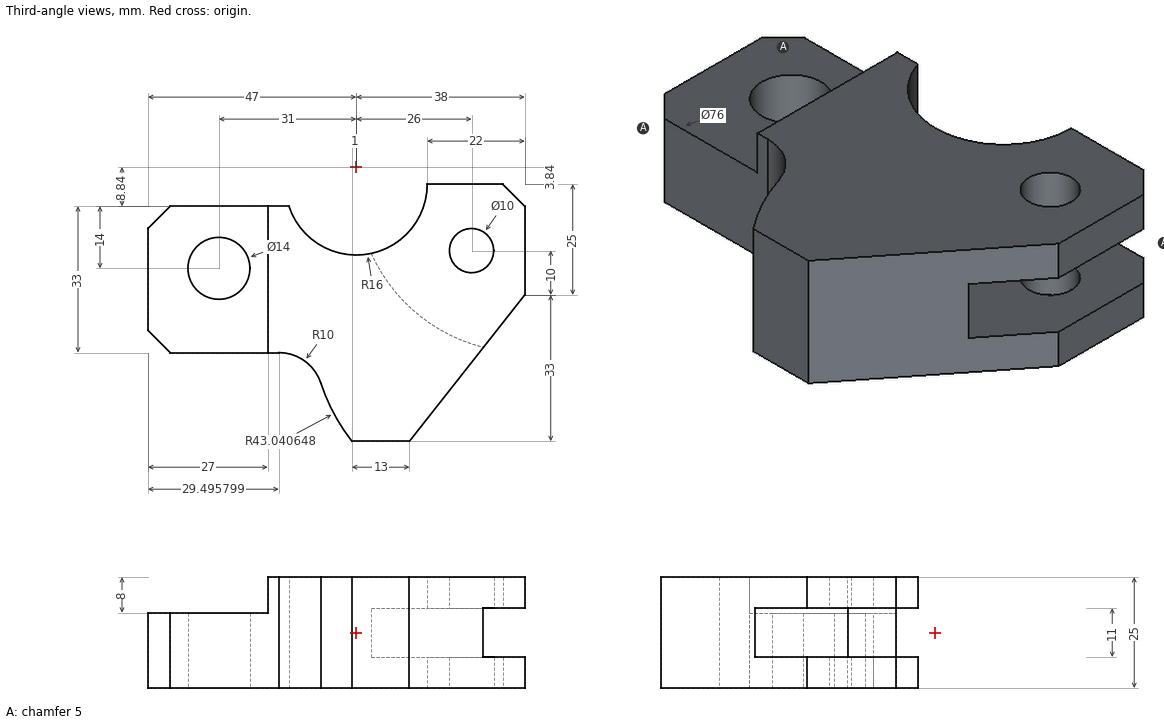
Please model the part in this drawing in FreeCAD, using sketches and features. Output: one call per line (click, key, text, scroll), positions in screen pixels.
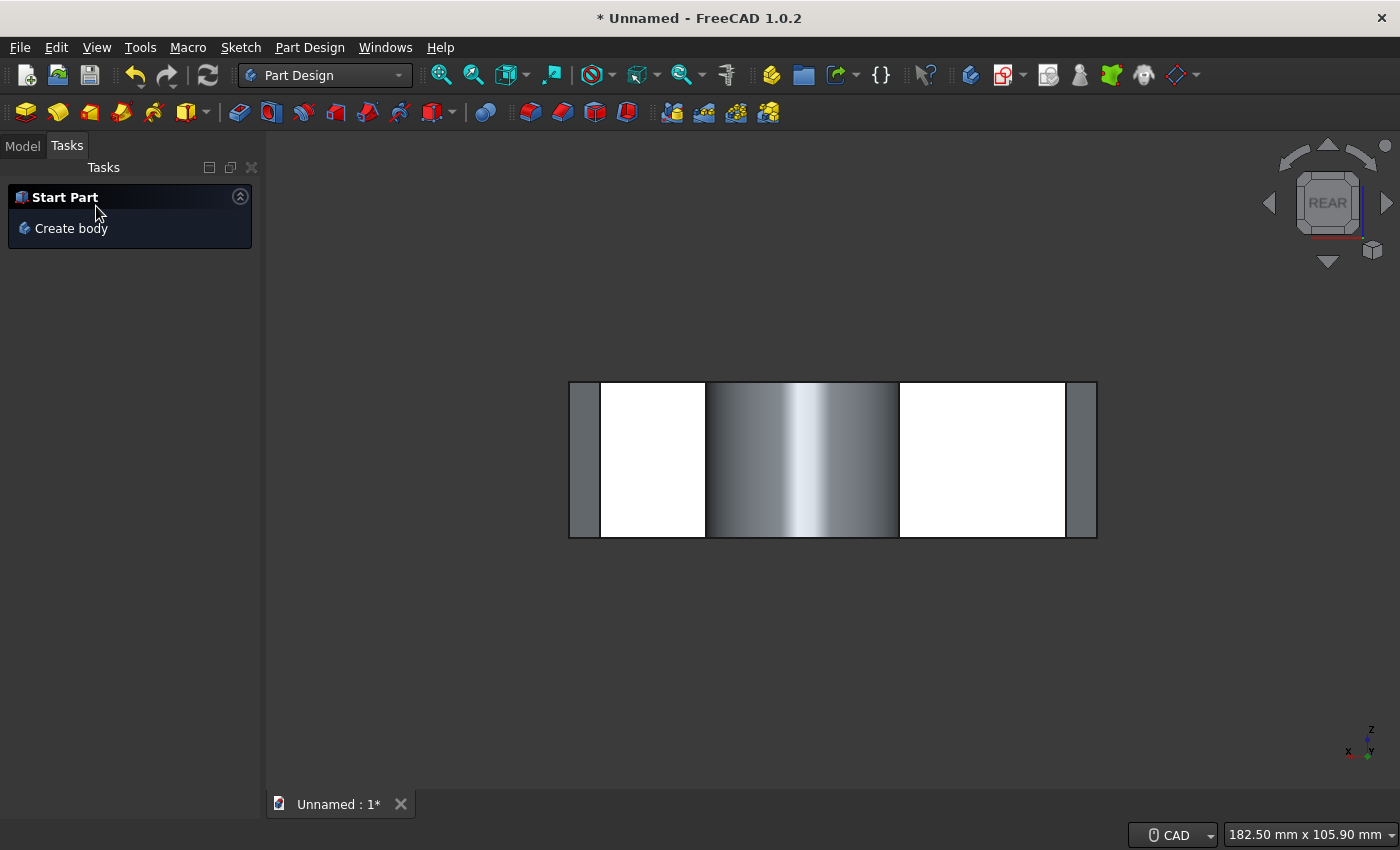
key(0)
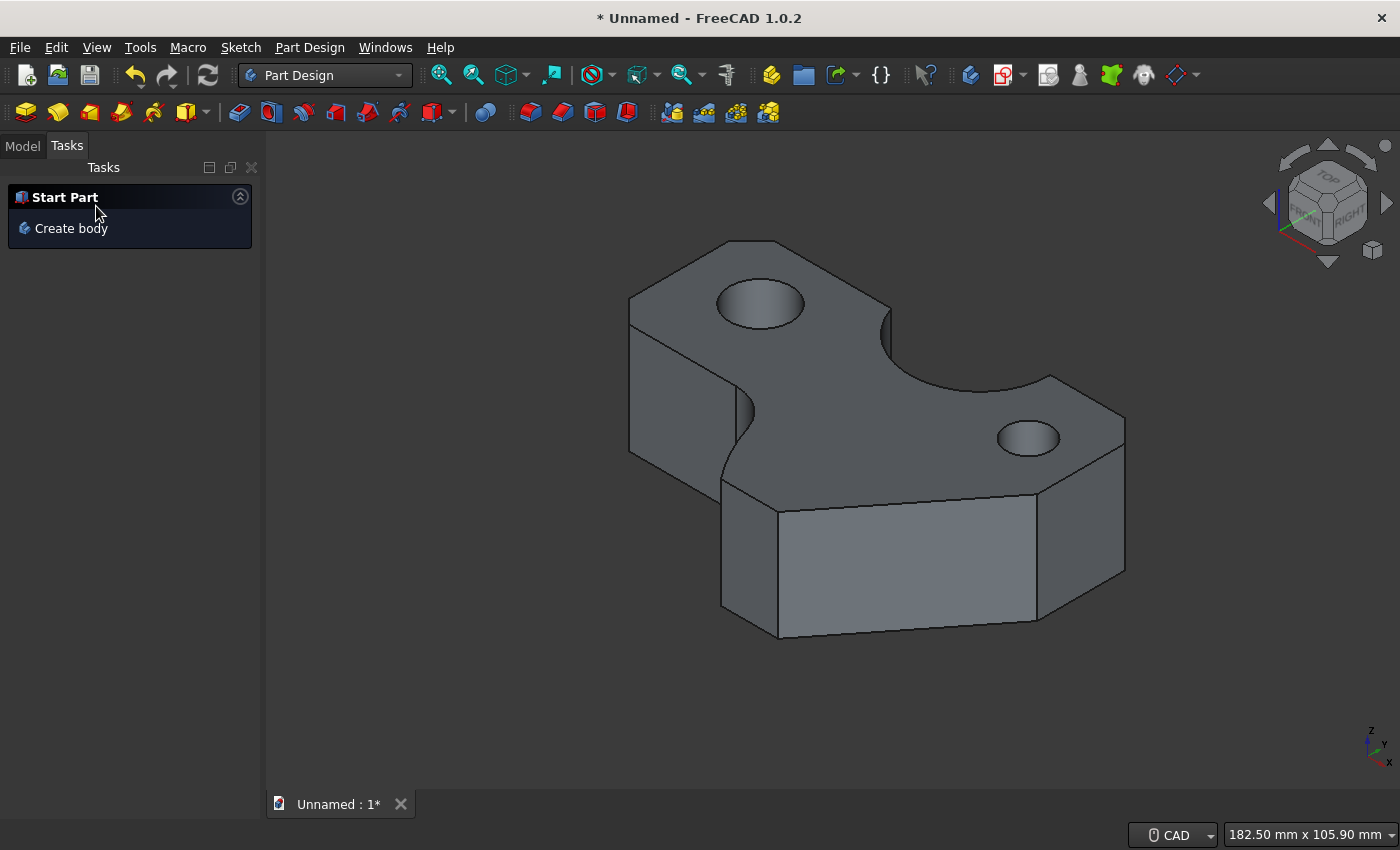
click(850, 447)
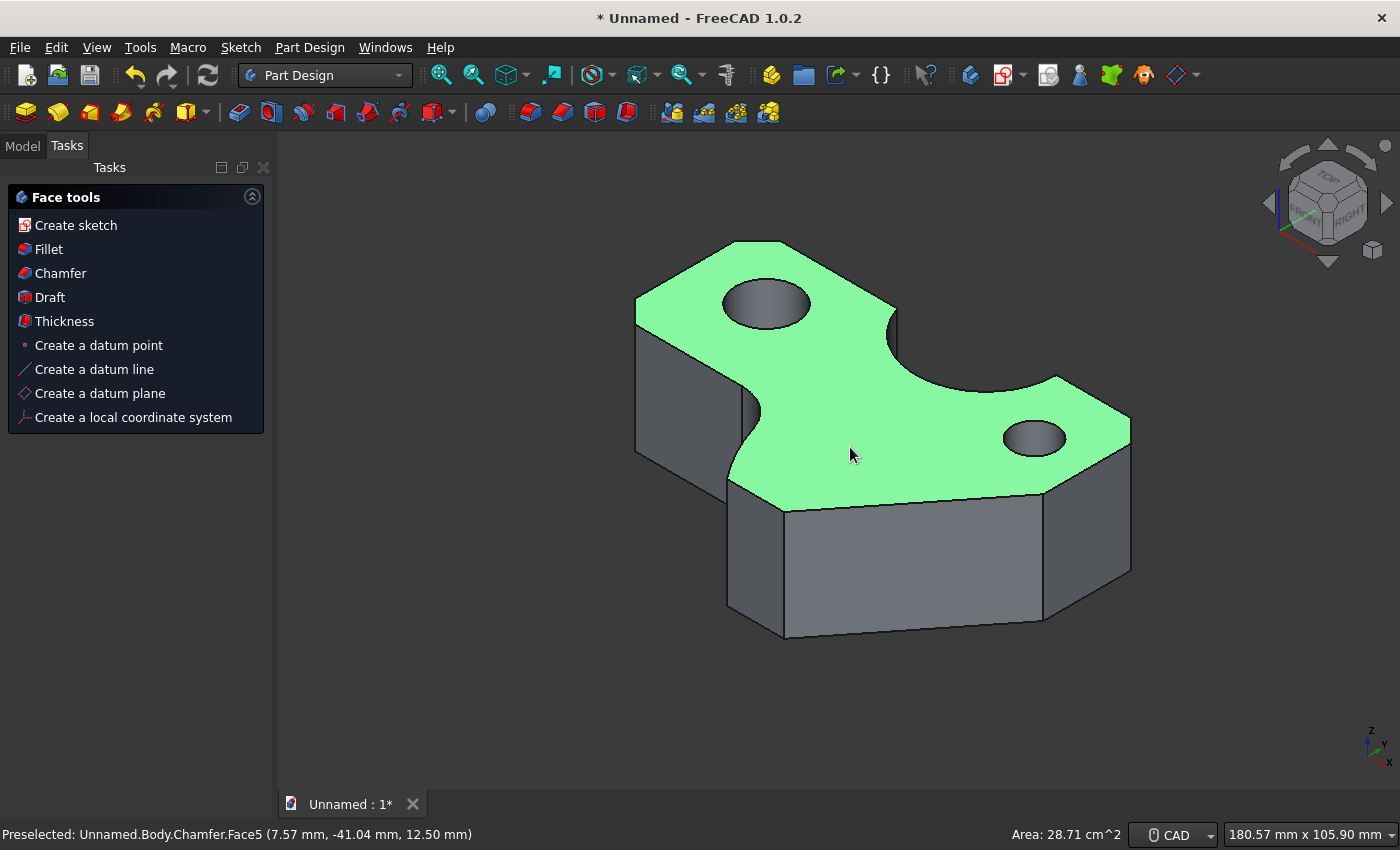
click(1004, 76)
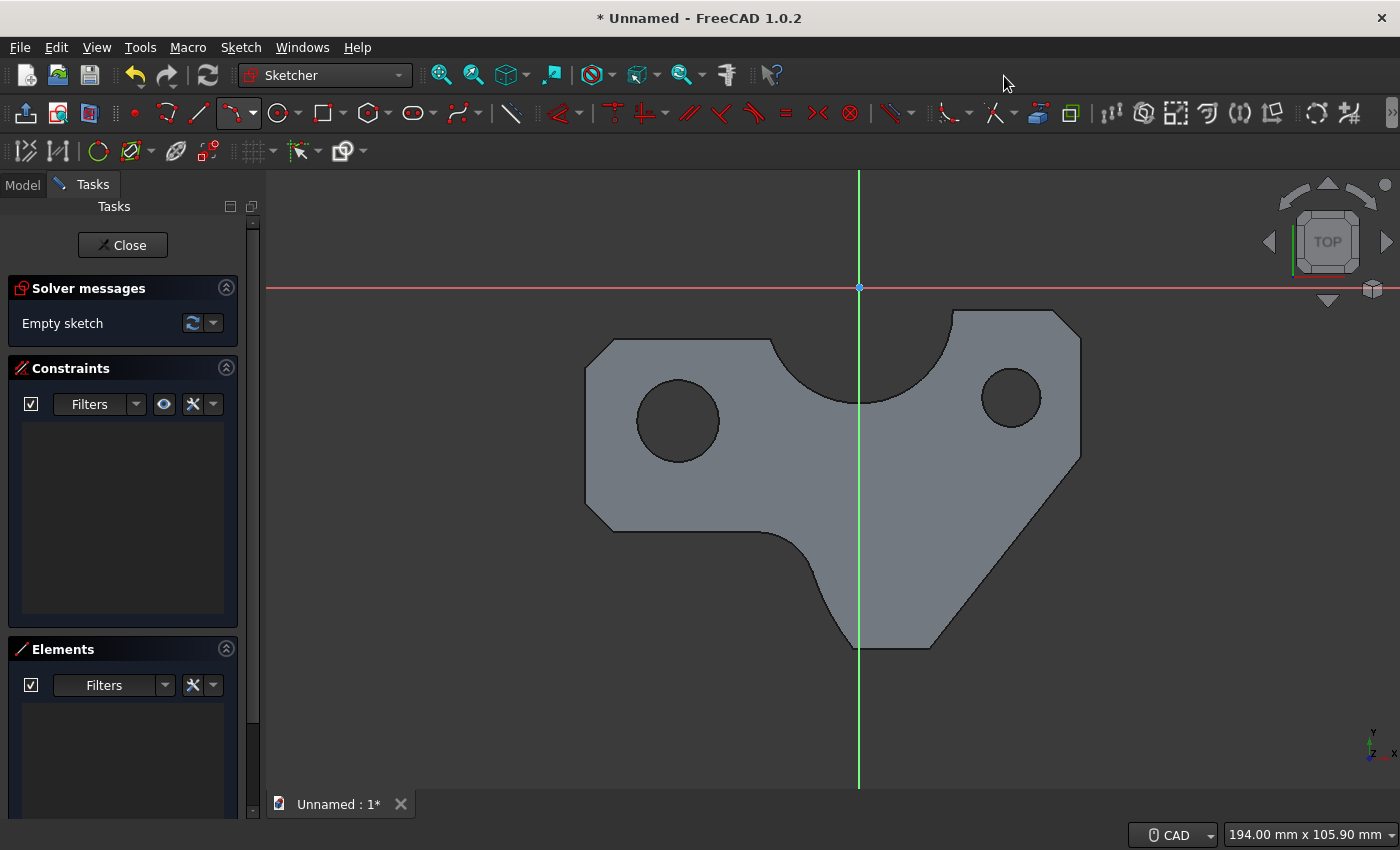
scroll(635, 268, up, 2)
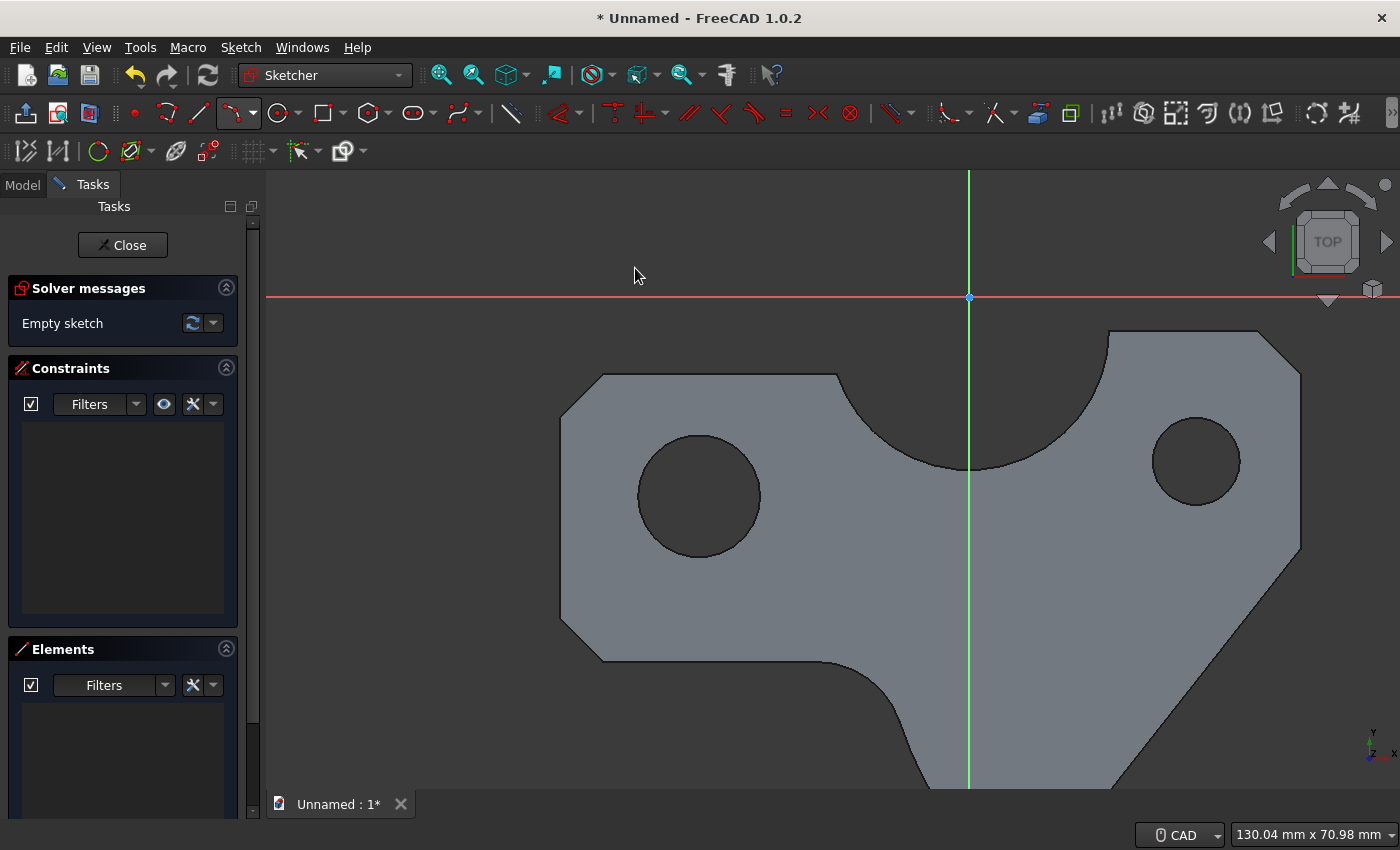
key(g)
key(r)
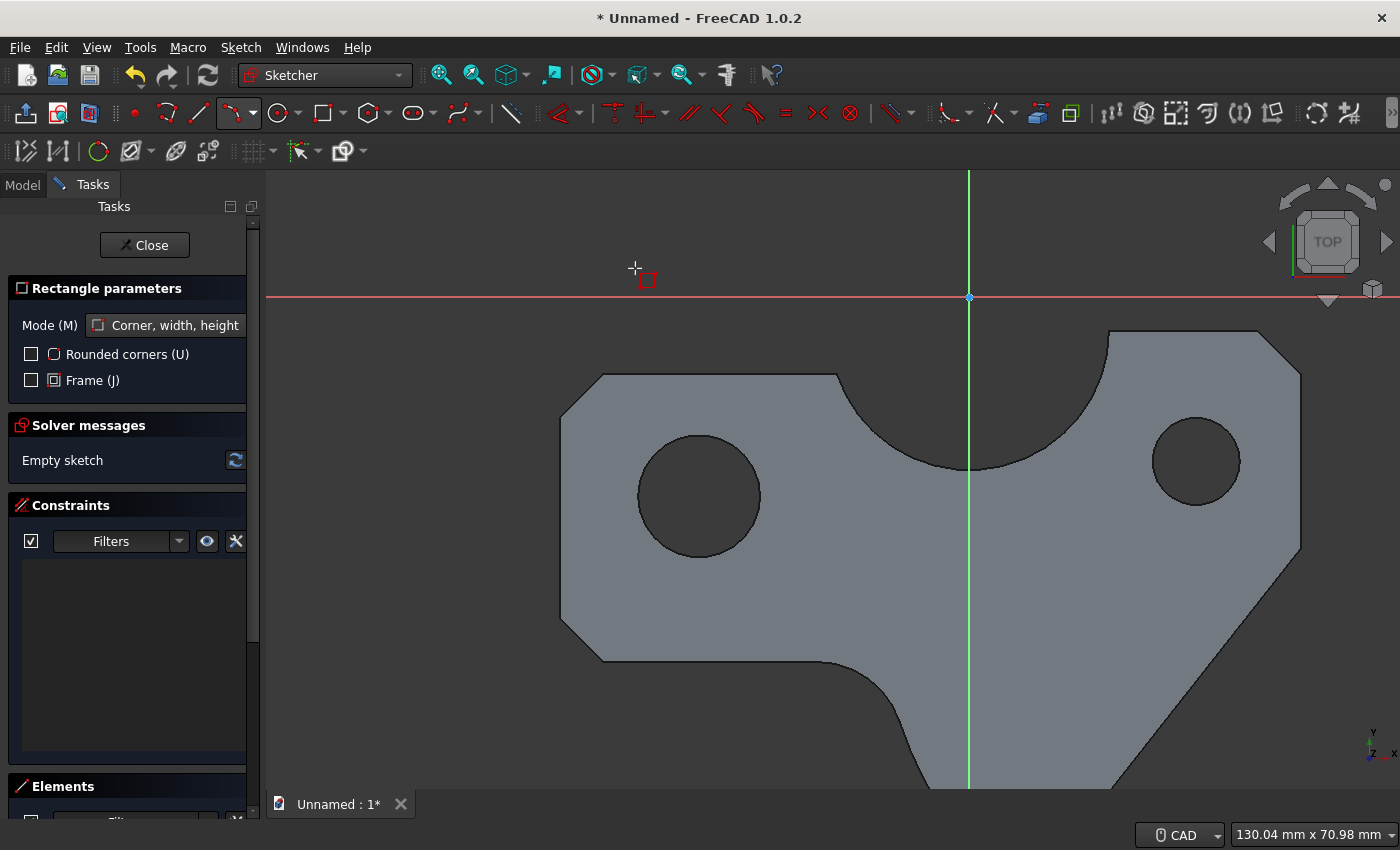
click(560, 374)
move(795, 662)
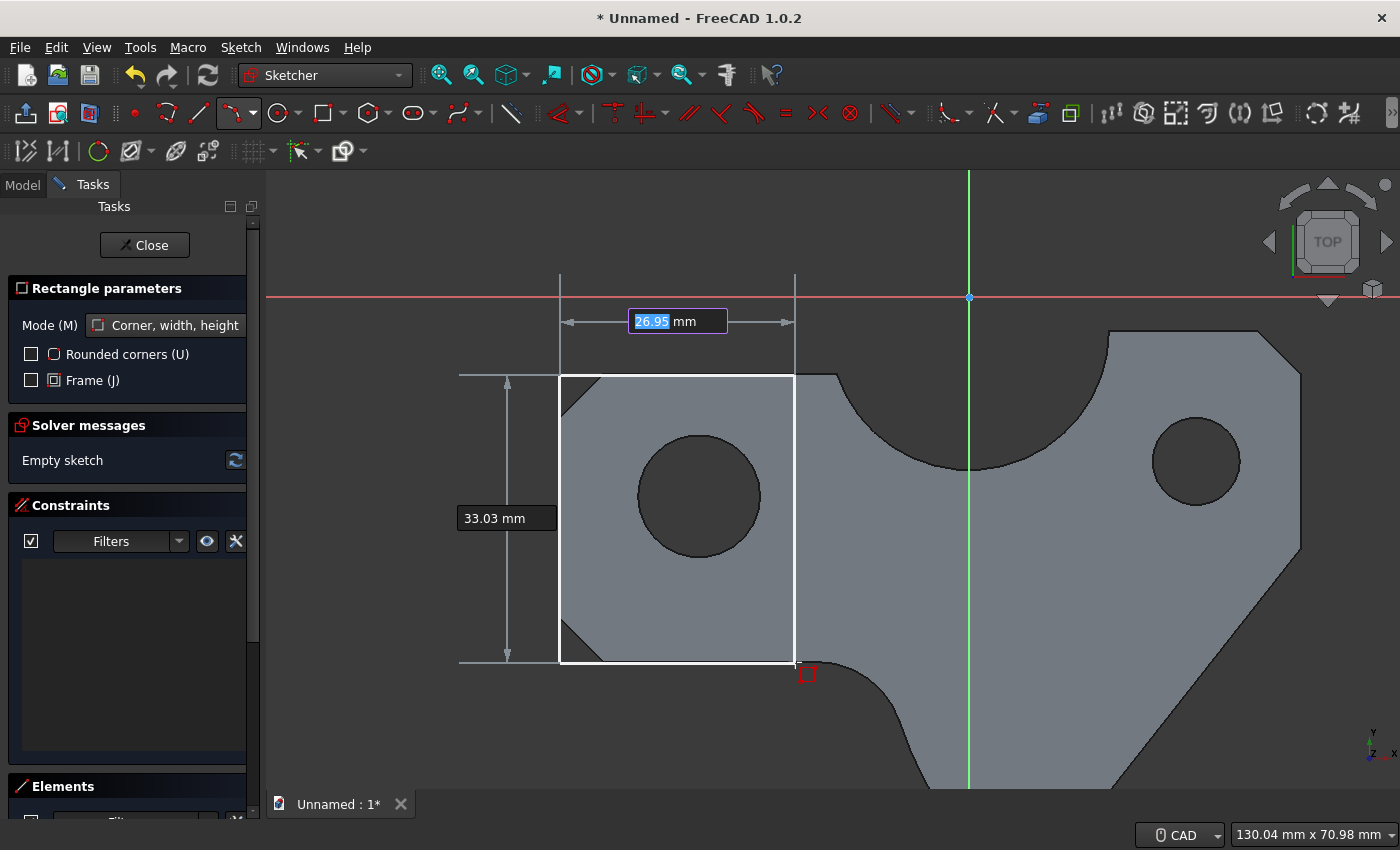
text(27)
key(Tab)
text(33)
key(Return)
key(Escape)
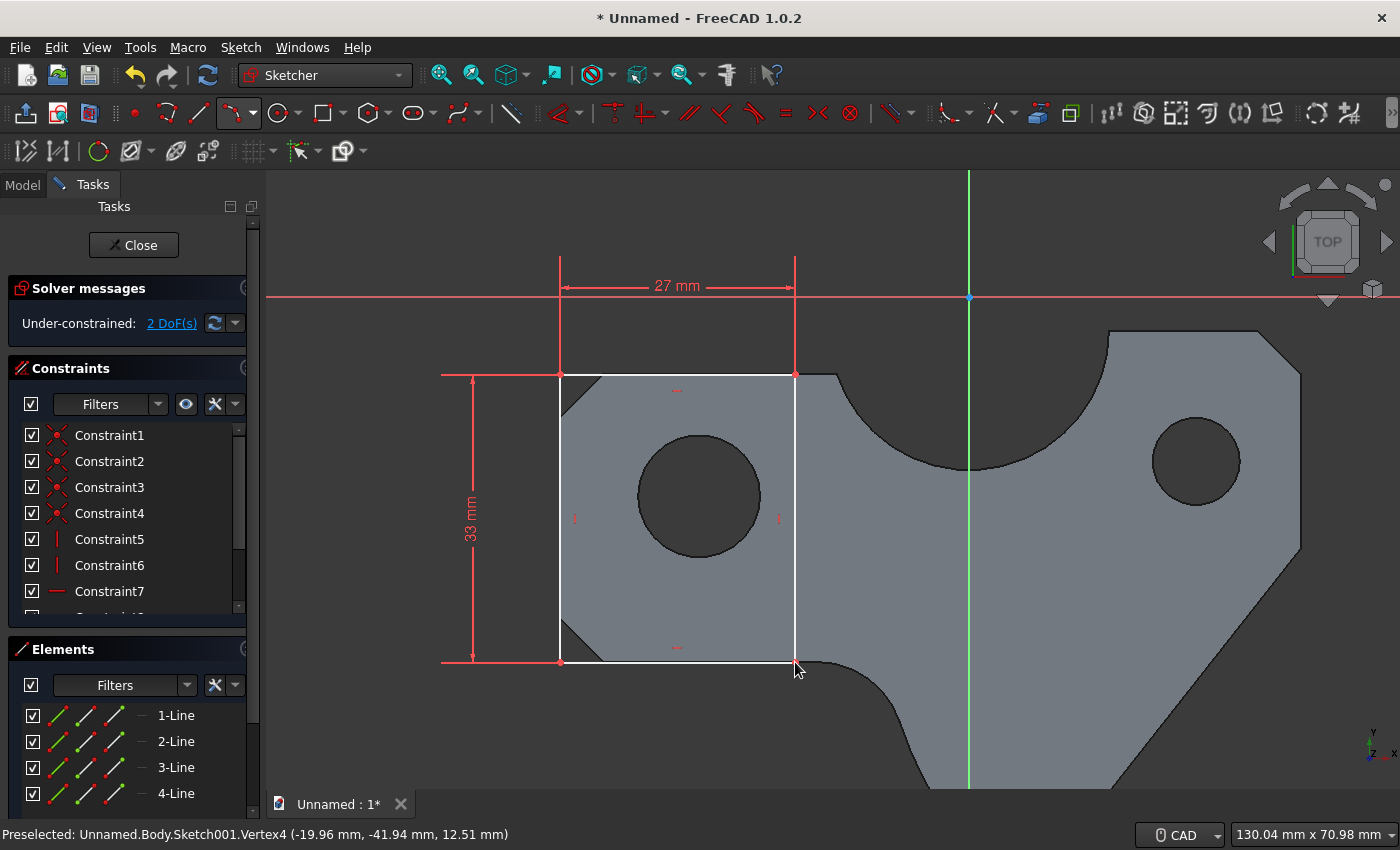
key(d)